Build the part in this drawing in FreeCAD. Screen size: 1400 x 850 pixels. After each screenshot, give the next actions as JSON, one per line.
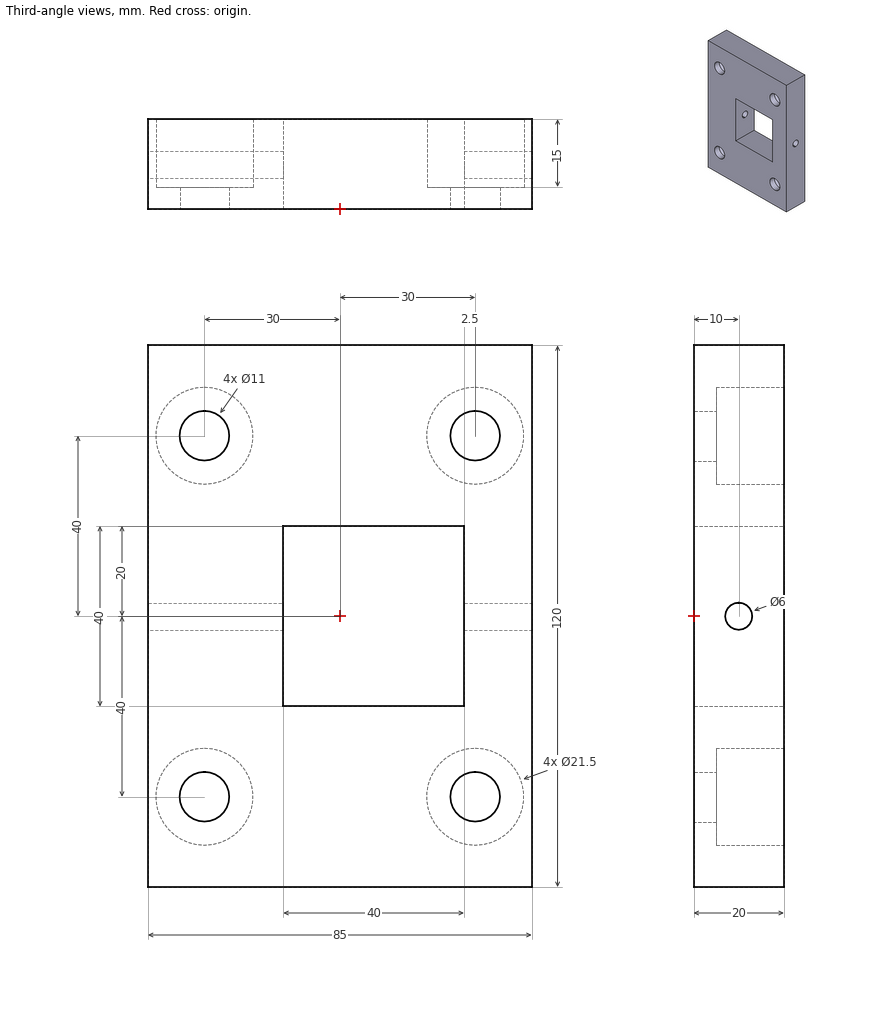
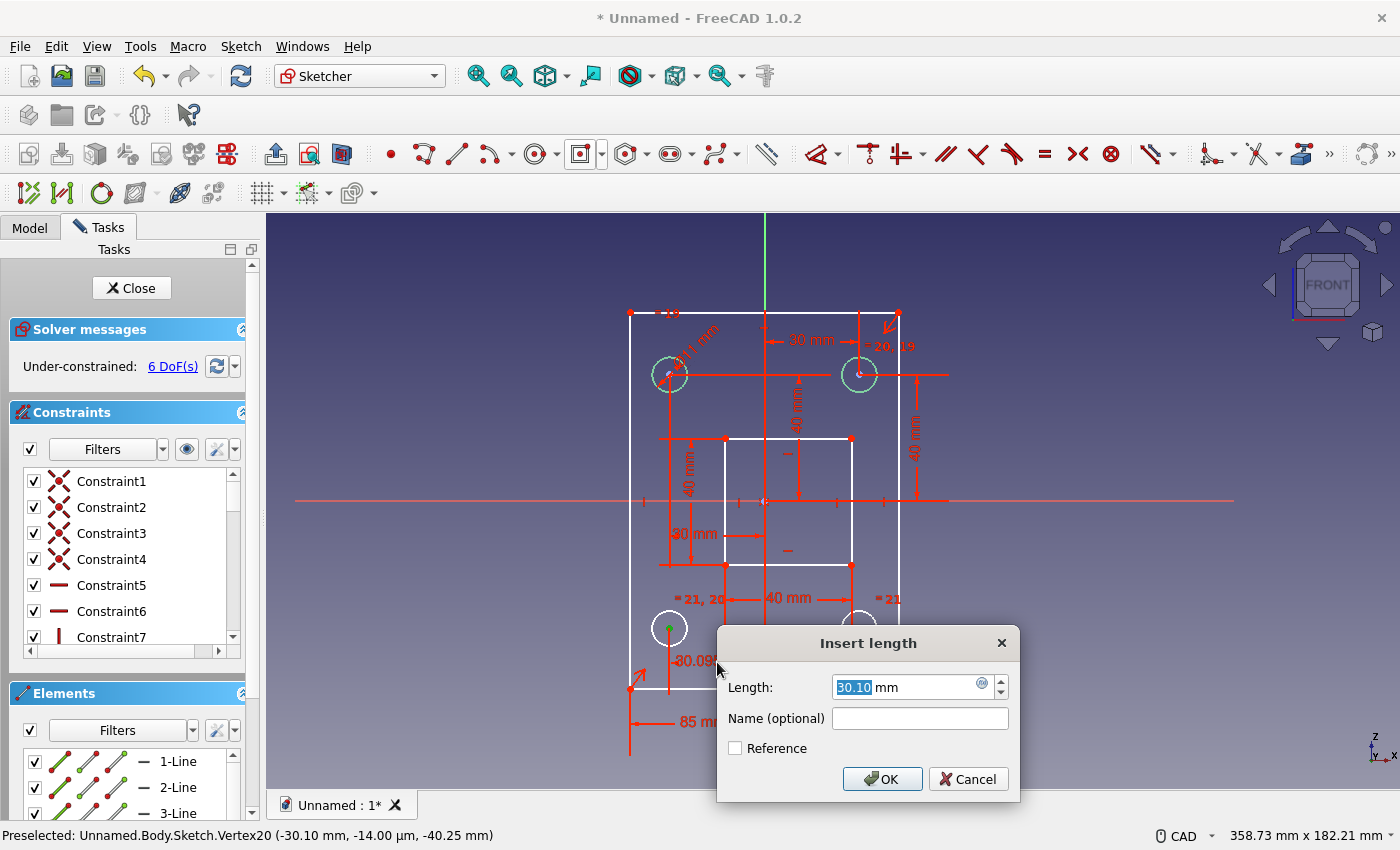
{"action": "type", "text": "30"}
{"action": "key", "text": "Return"}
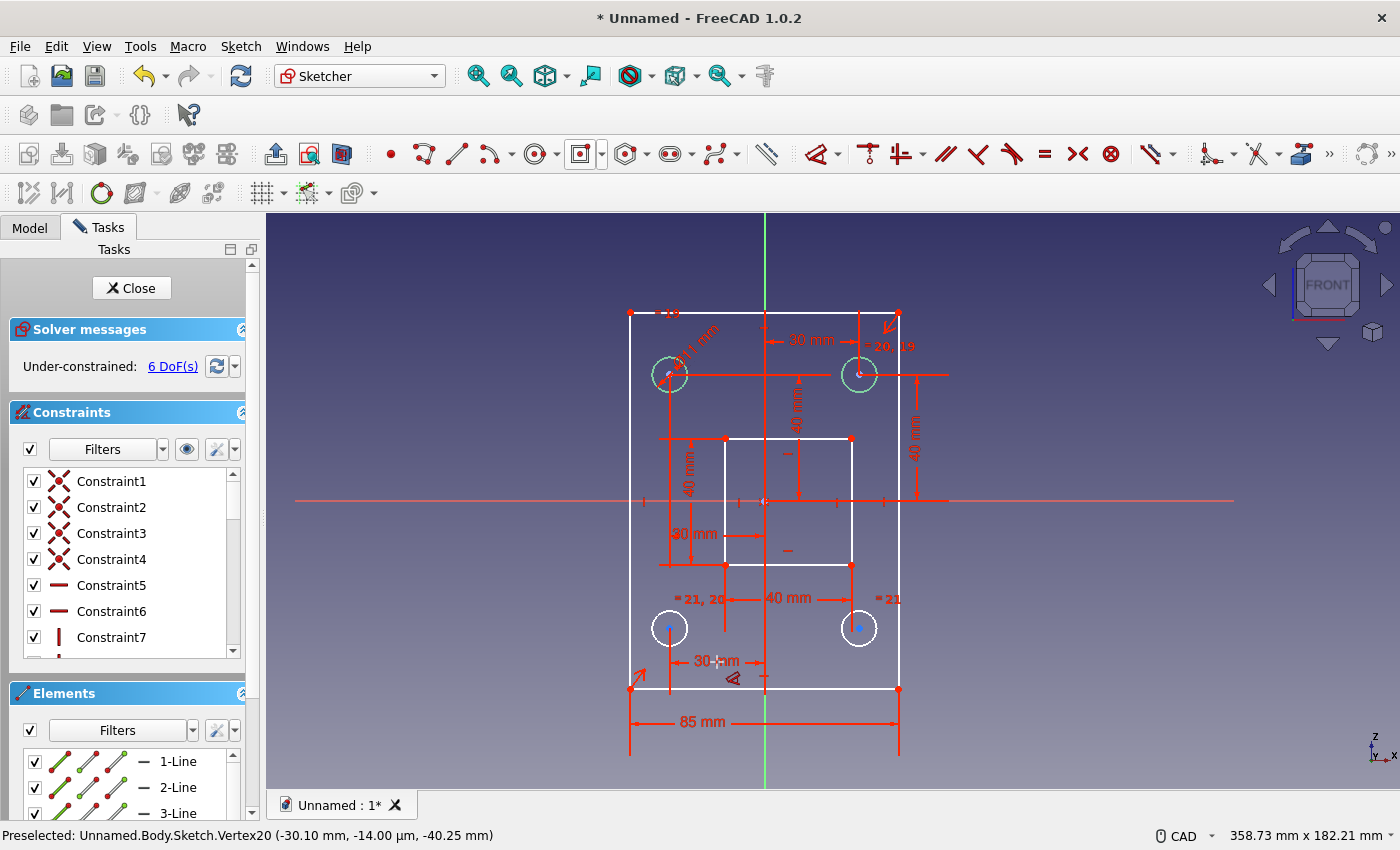
{"action": "left_click", "coordinate": [670, 628]}
{"action": "left_click", "coordinate": [799, 536]}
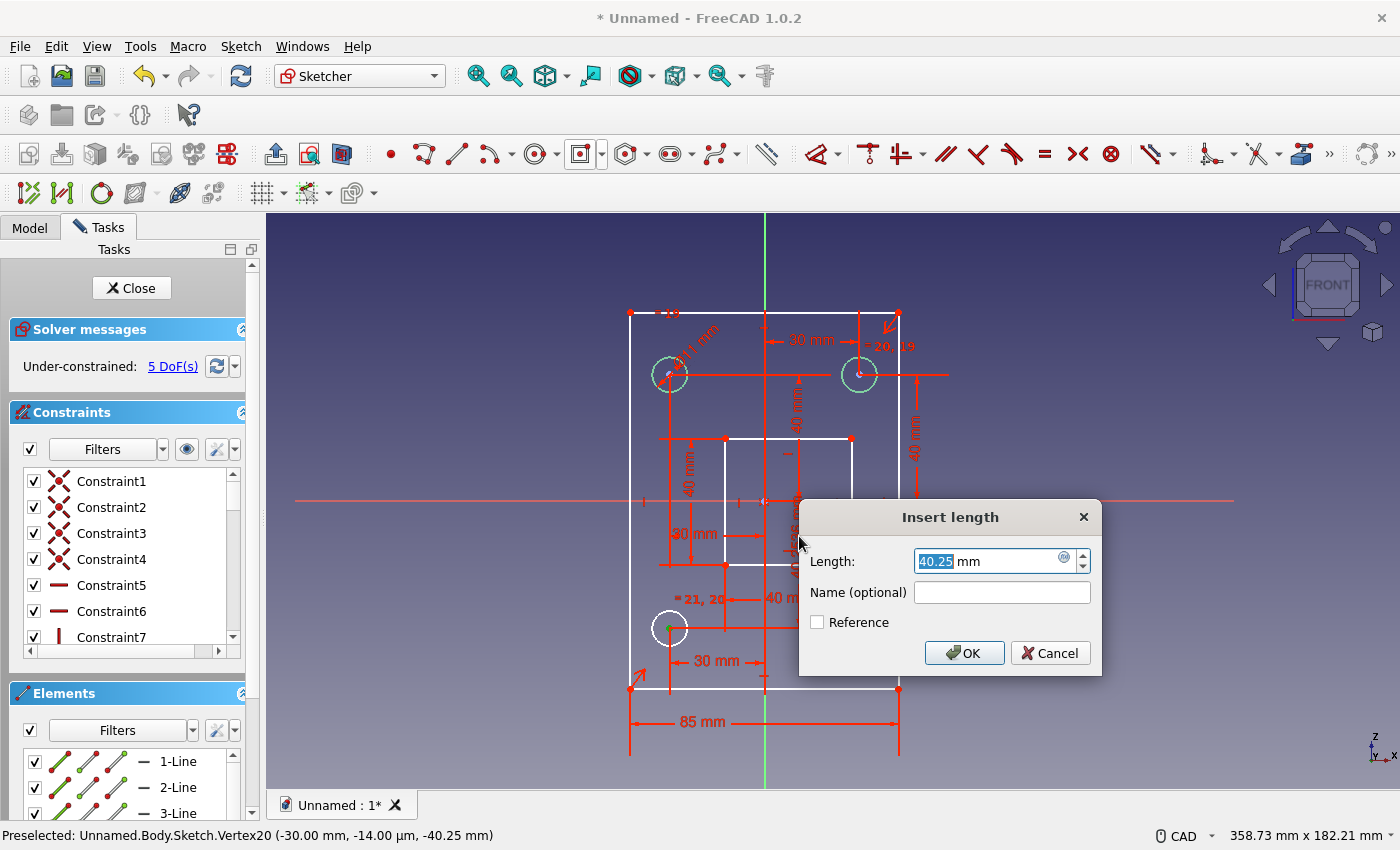
{"action": "type", "text": "40"}
{"action": "key", "text": "Return"}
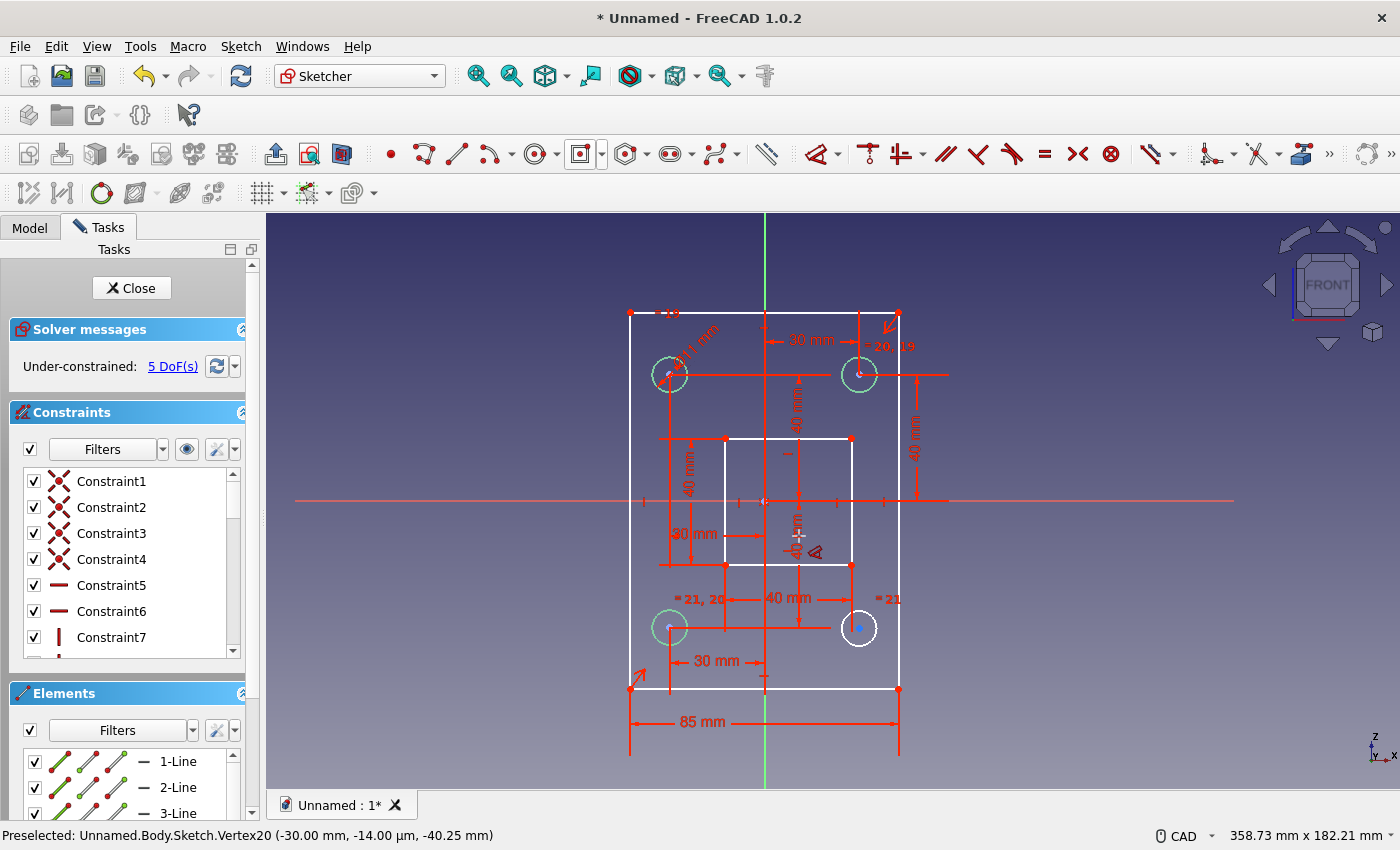
{"action": "left_click", "coordinate": [859, 628]}
{"action": "left_click", "coordinate": [812, 662]}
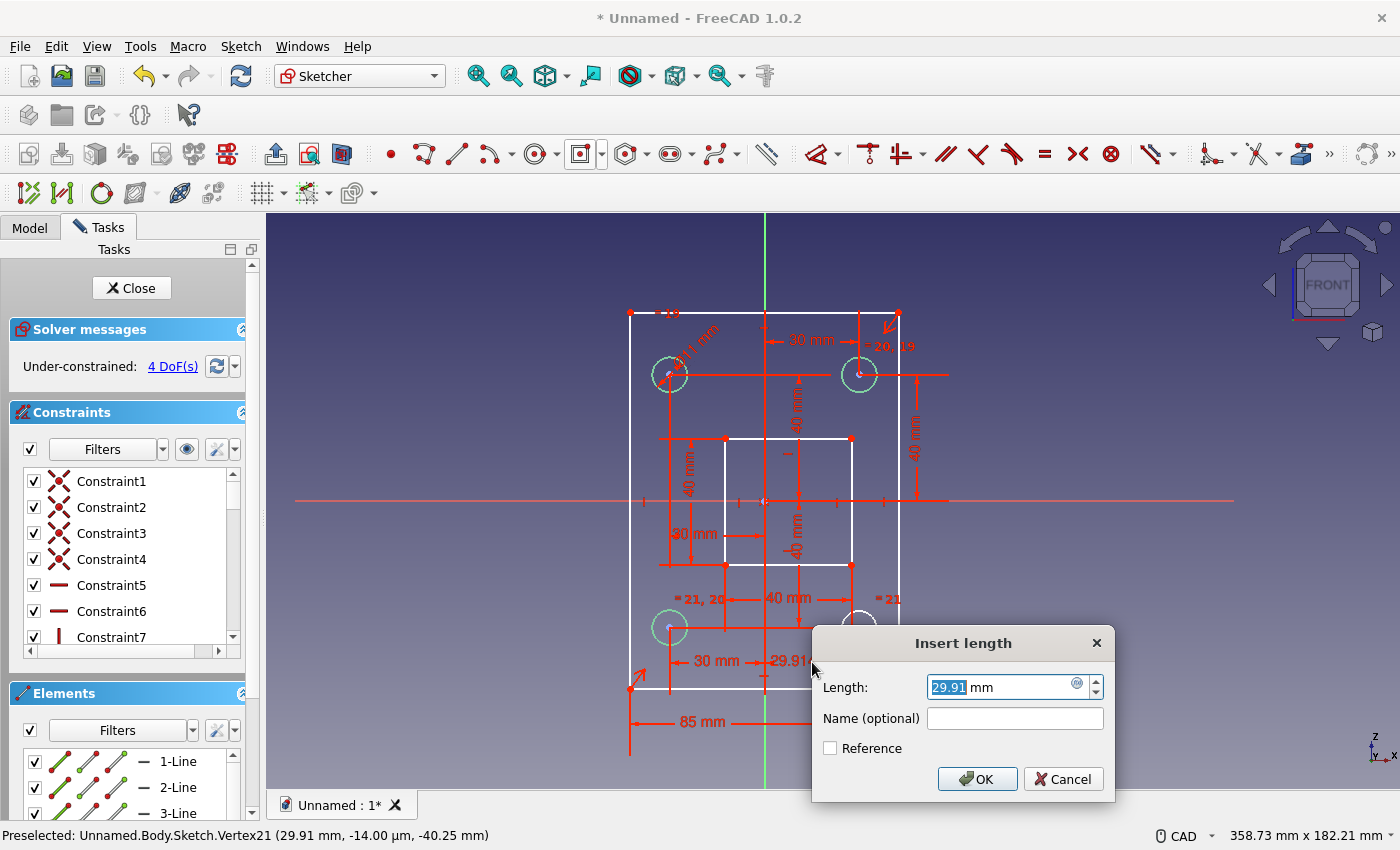
{"action": "type", "text": "30"}
{"action": "key", "text": "Return"}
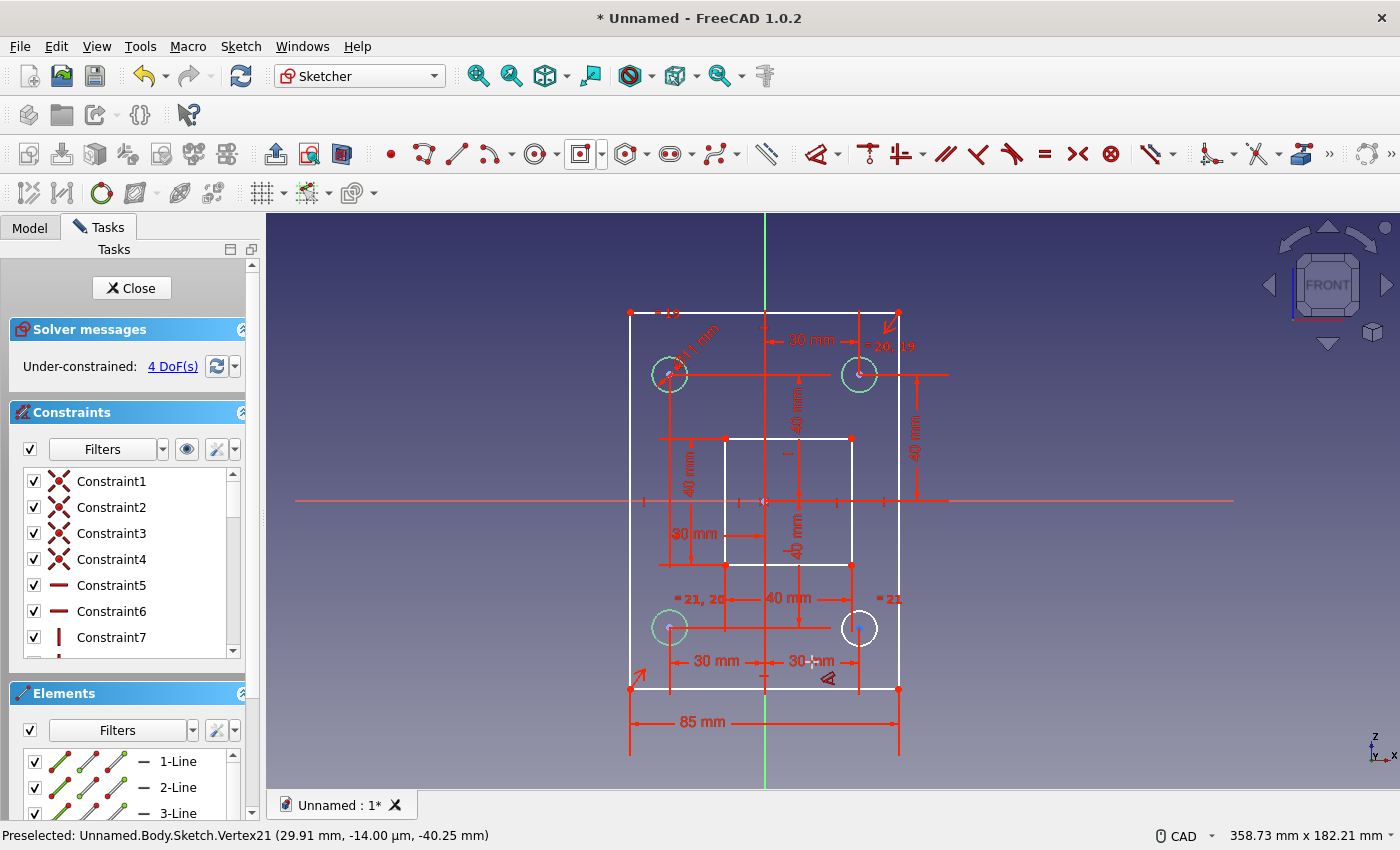
{"action": "left_click", "coordinate": [859, 628]}
{"action": "left_click", "coordinate": [917, 565]}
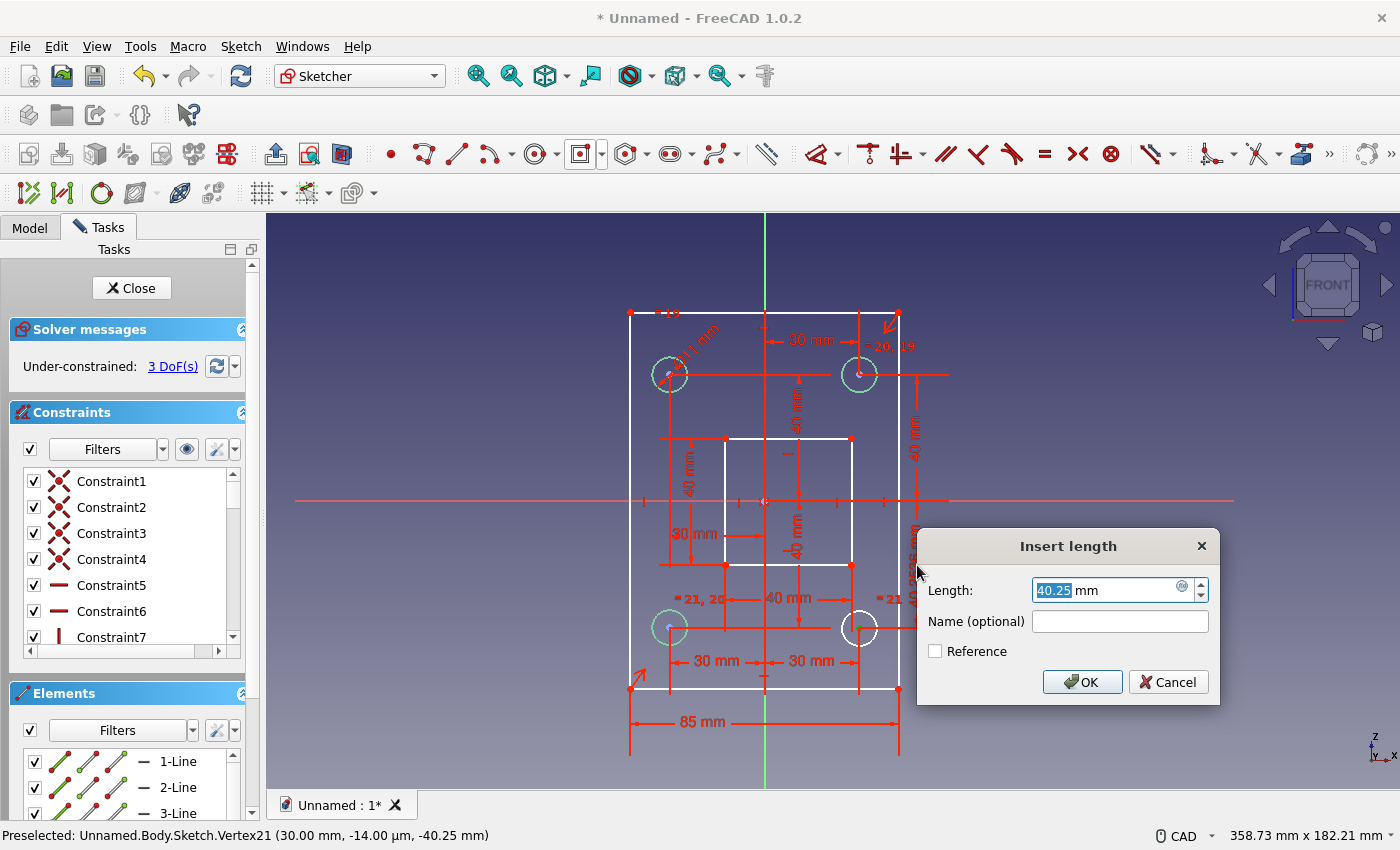
{"action": "type", "text": "40"}
{"action": "key", "text": "Return"}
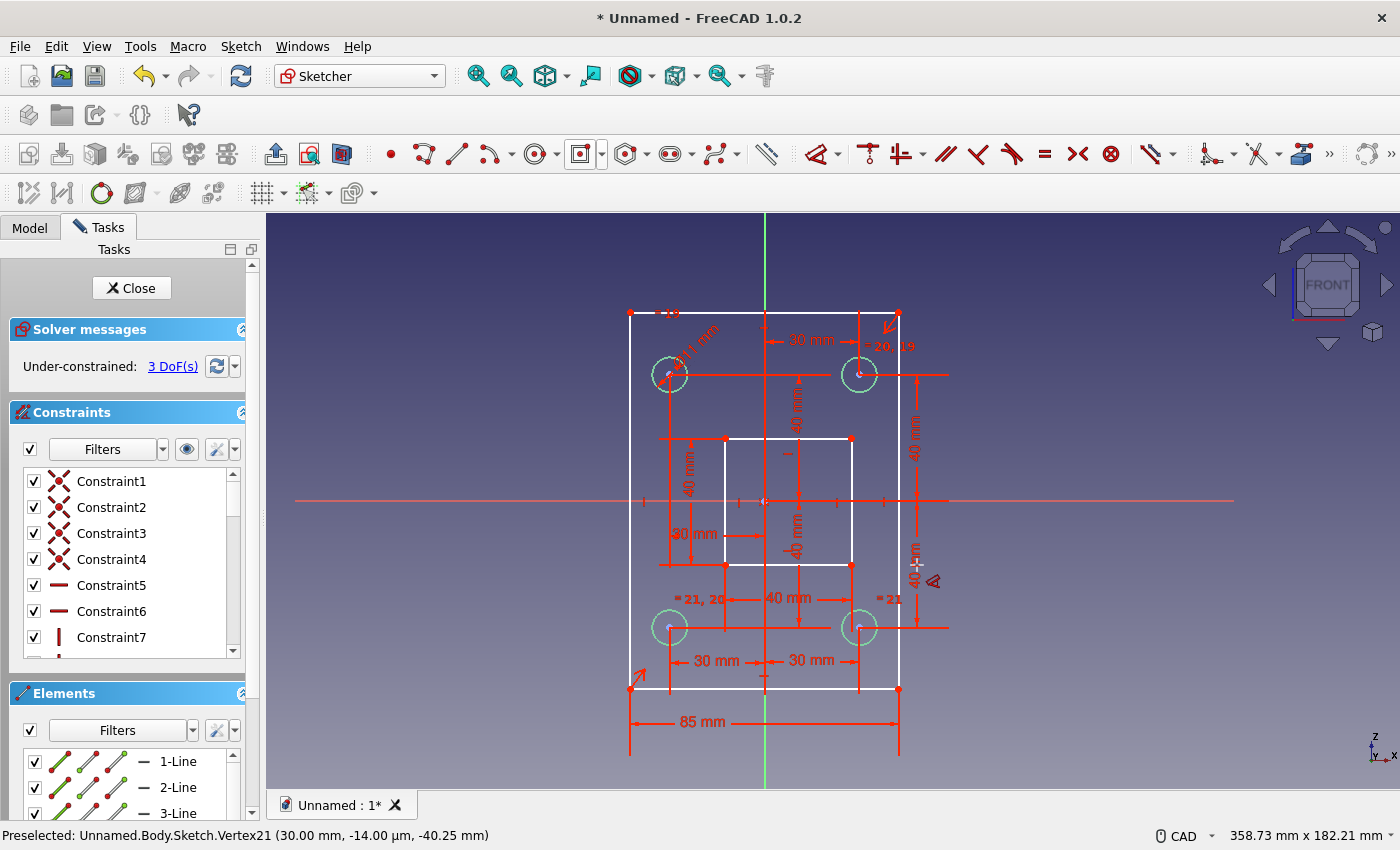
{"action": "left_click", "coordinate": [899, 577]}
{"action": "left_click", "coordinate": [933, 415]}